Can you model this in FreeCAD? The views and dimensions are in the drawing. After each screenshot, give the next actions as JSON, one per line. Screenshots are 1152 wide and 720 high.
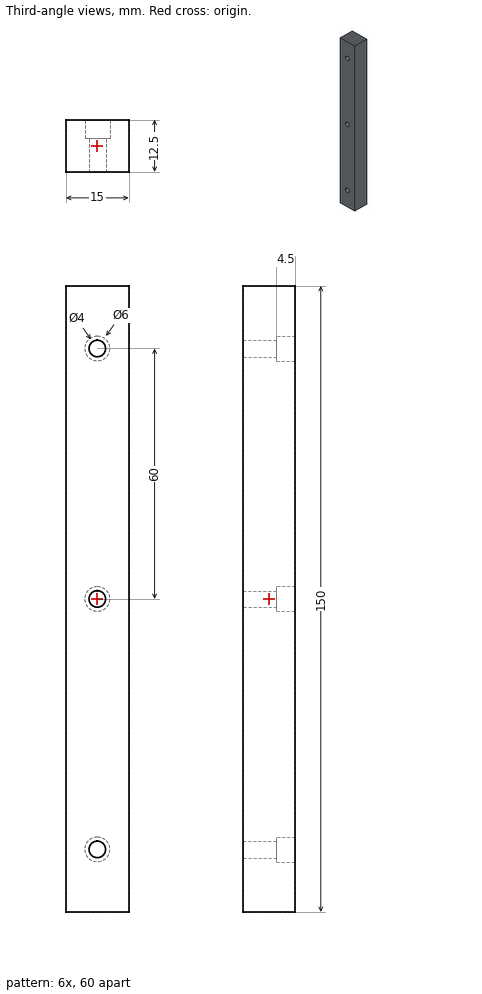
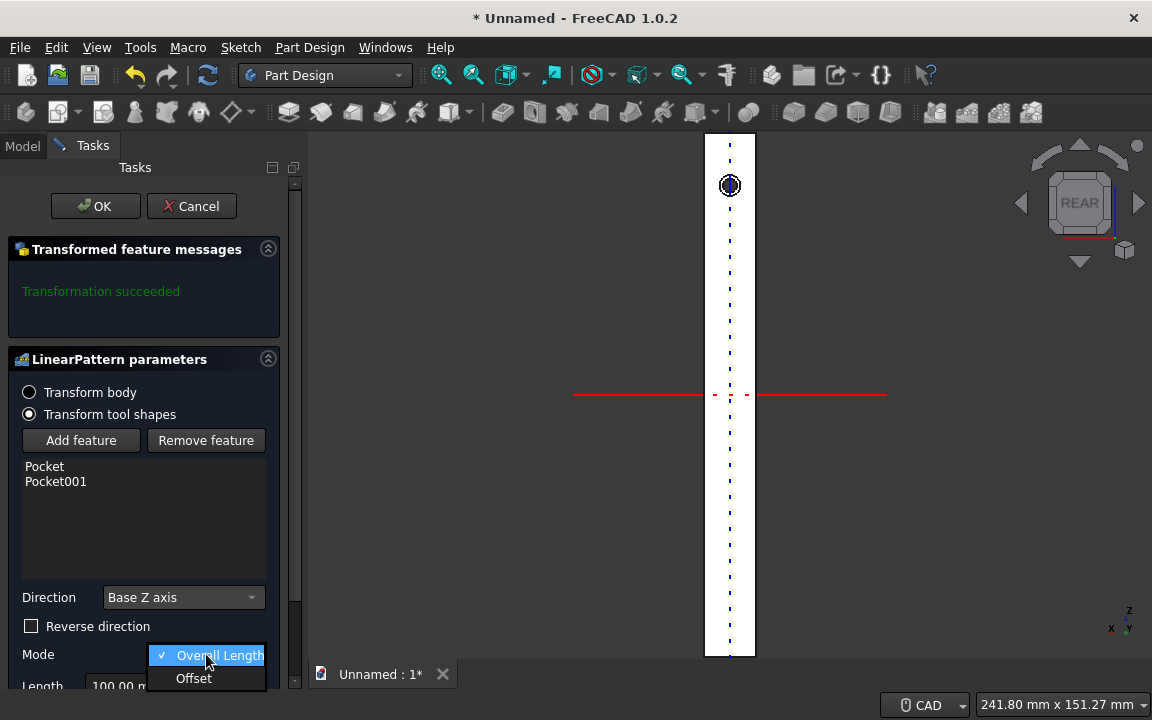
{"action": "left_click", "coordinate": [206, 678]}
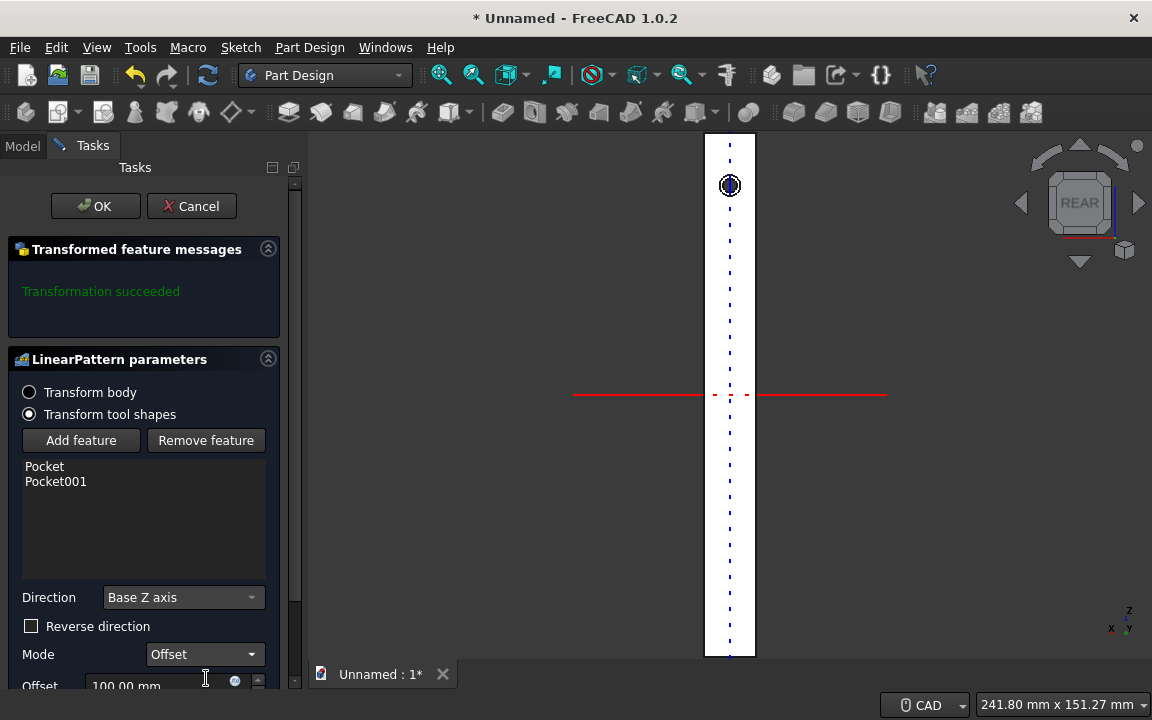
{"action": "scroll", "coordinate": [295, 432], "scroll_direction": "down", "scroll_amount": 2}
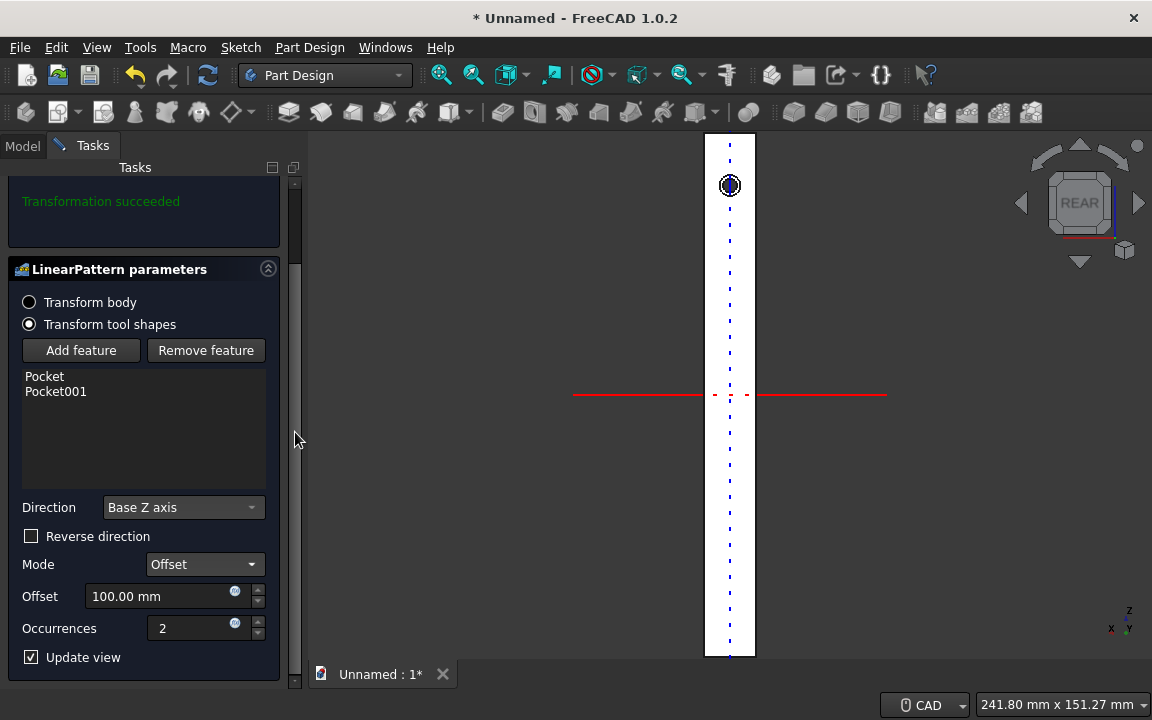
{"action": "triple_click", "coordinate": [168, 596]}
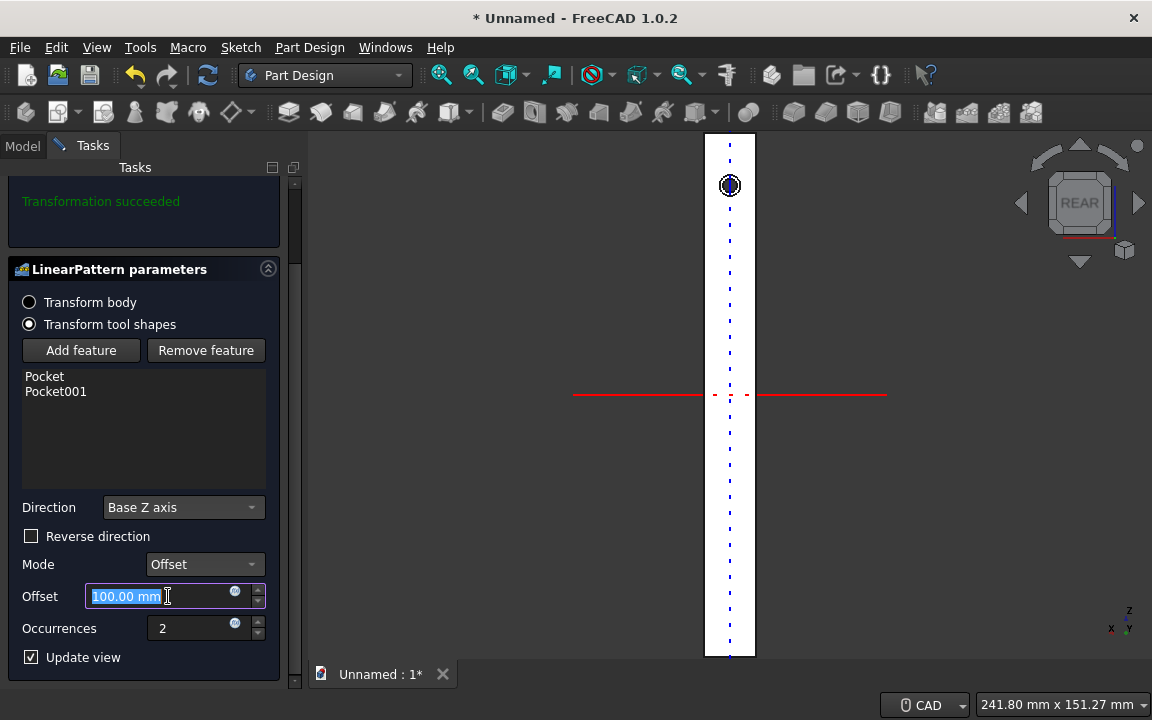
{"action": "type", "text": "60"}
{"action": "key", "text": "Tab"}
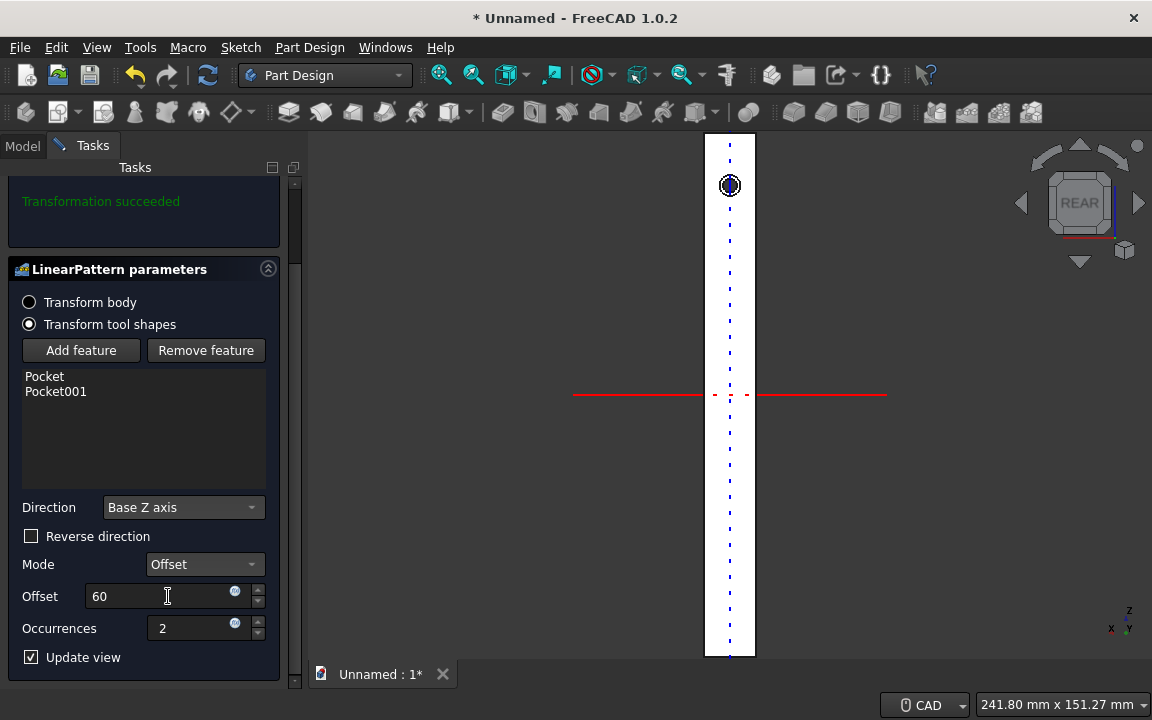
{"action": "triple_click", "coordinate": [198, 628]}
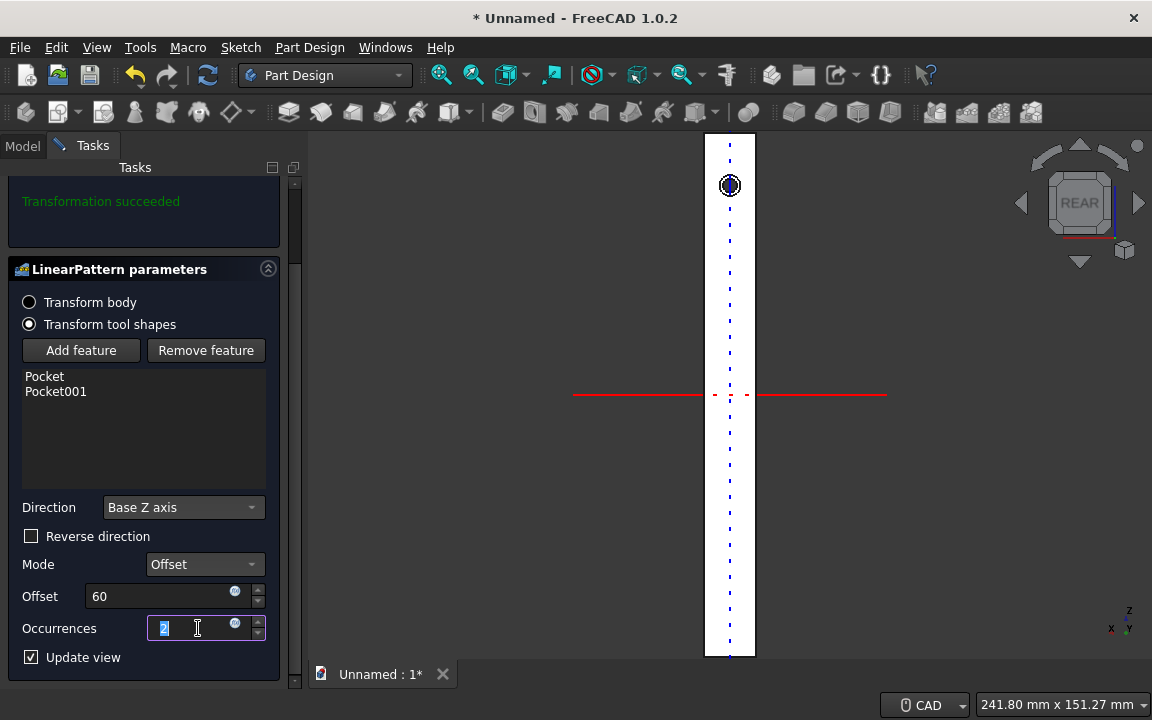
{"action": "type", "text": "6"}
{"action": "key", "text": "Tab"}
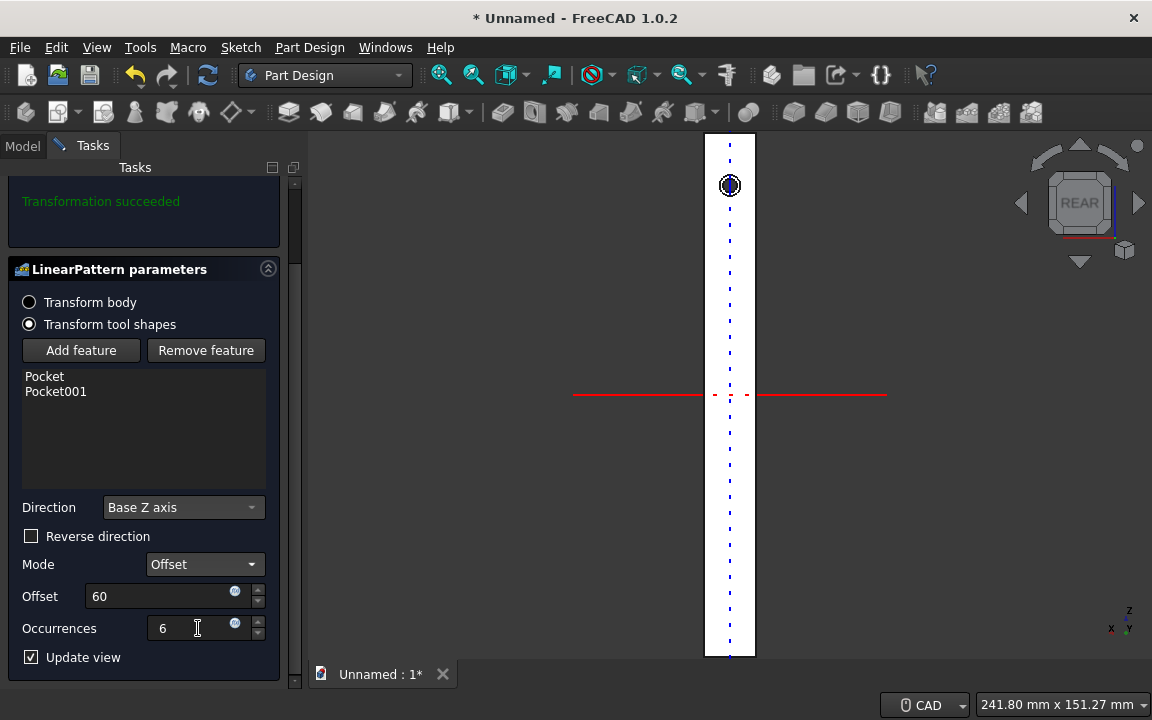
{"action": "left_click", "coordinate": [30, 536]}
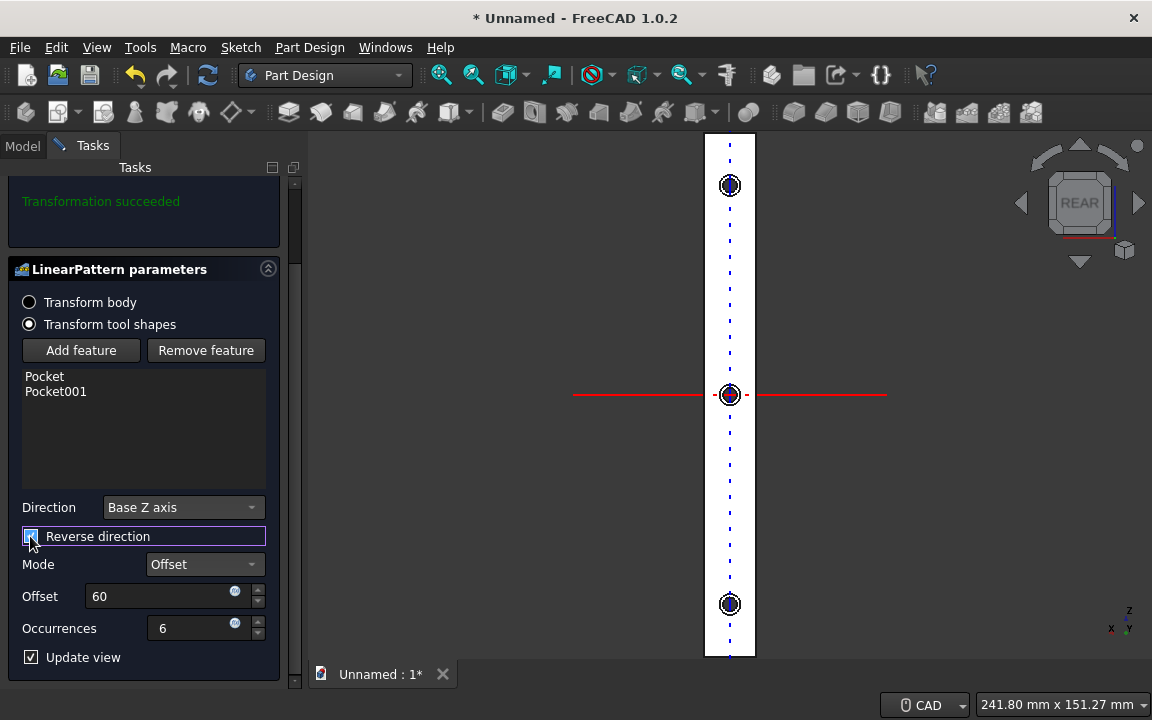
{"action": "scroll", "coordinate": [295, 432], "scroll_direction": "up", "scroll_amount": 3}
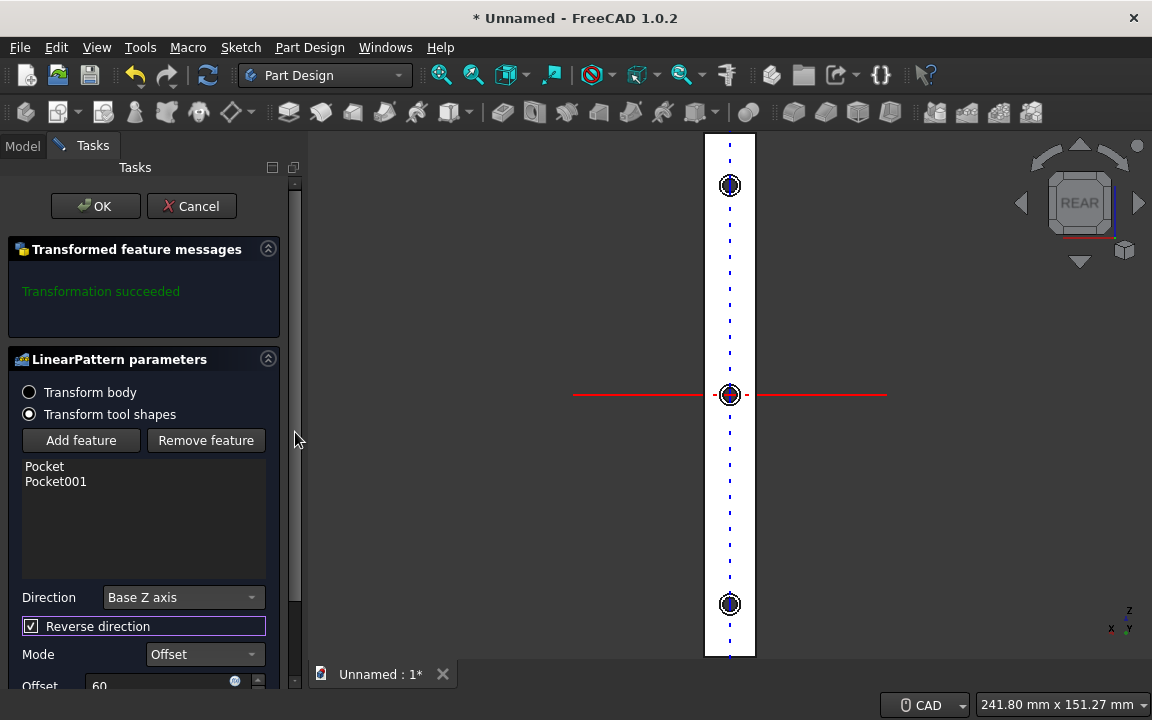
{"action": "left_click", "coordinate": [96, 206]}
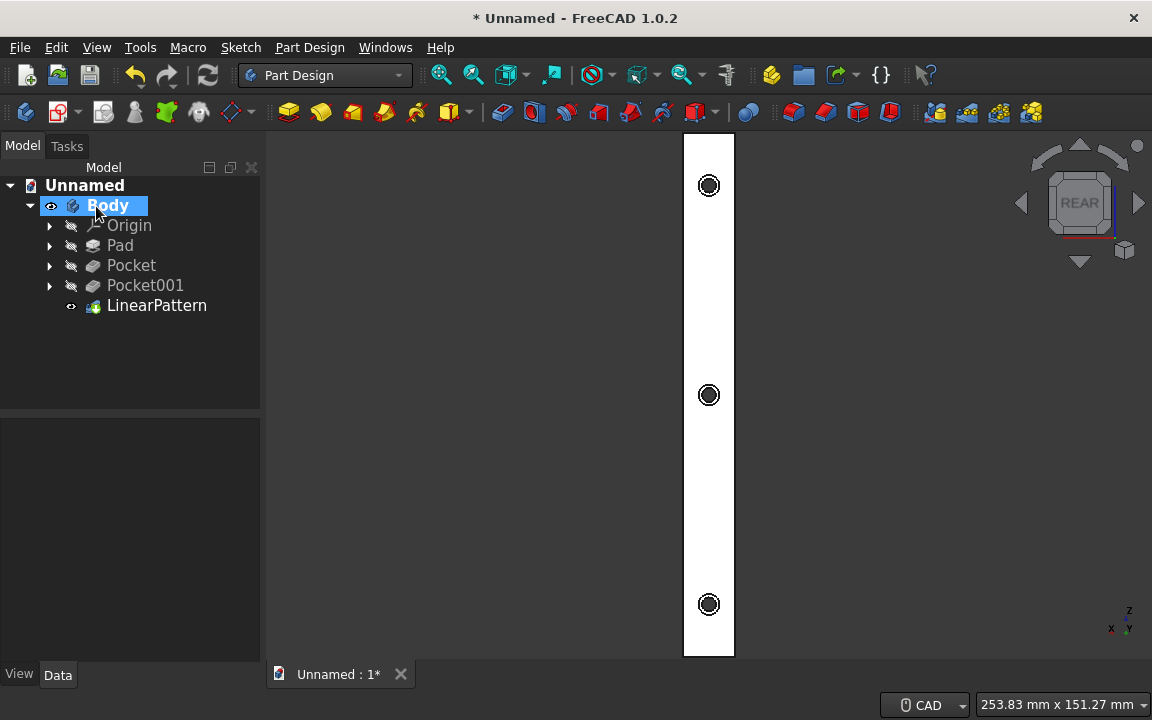
{"action": "key", "text": "0"}